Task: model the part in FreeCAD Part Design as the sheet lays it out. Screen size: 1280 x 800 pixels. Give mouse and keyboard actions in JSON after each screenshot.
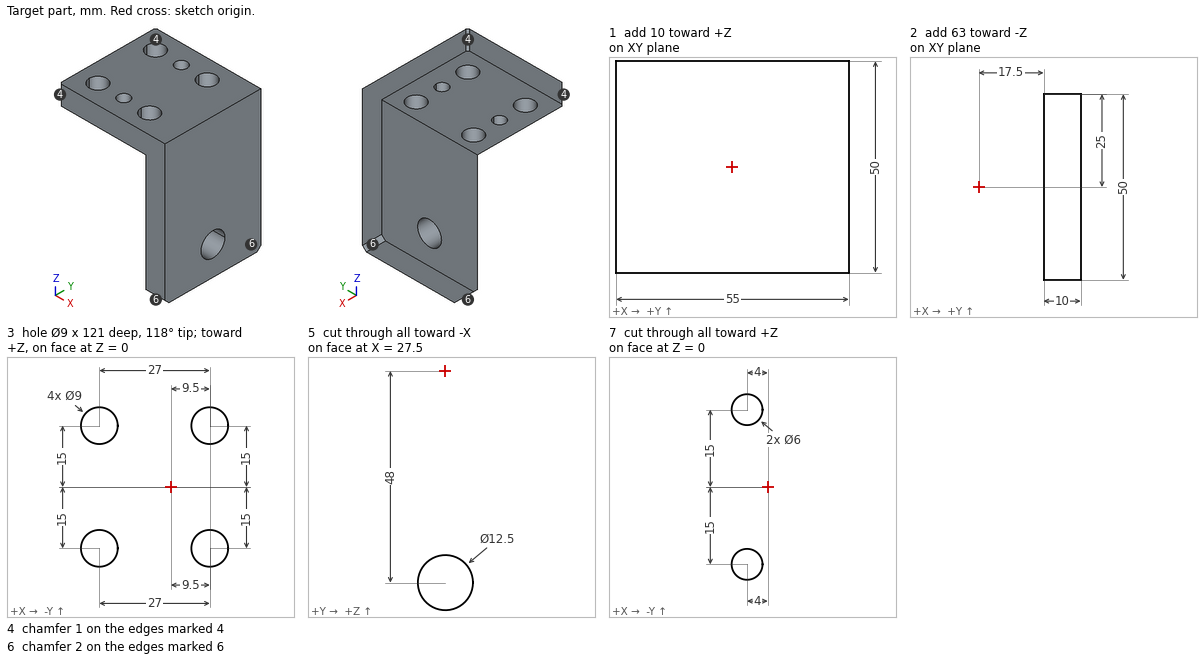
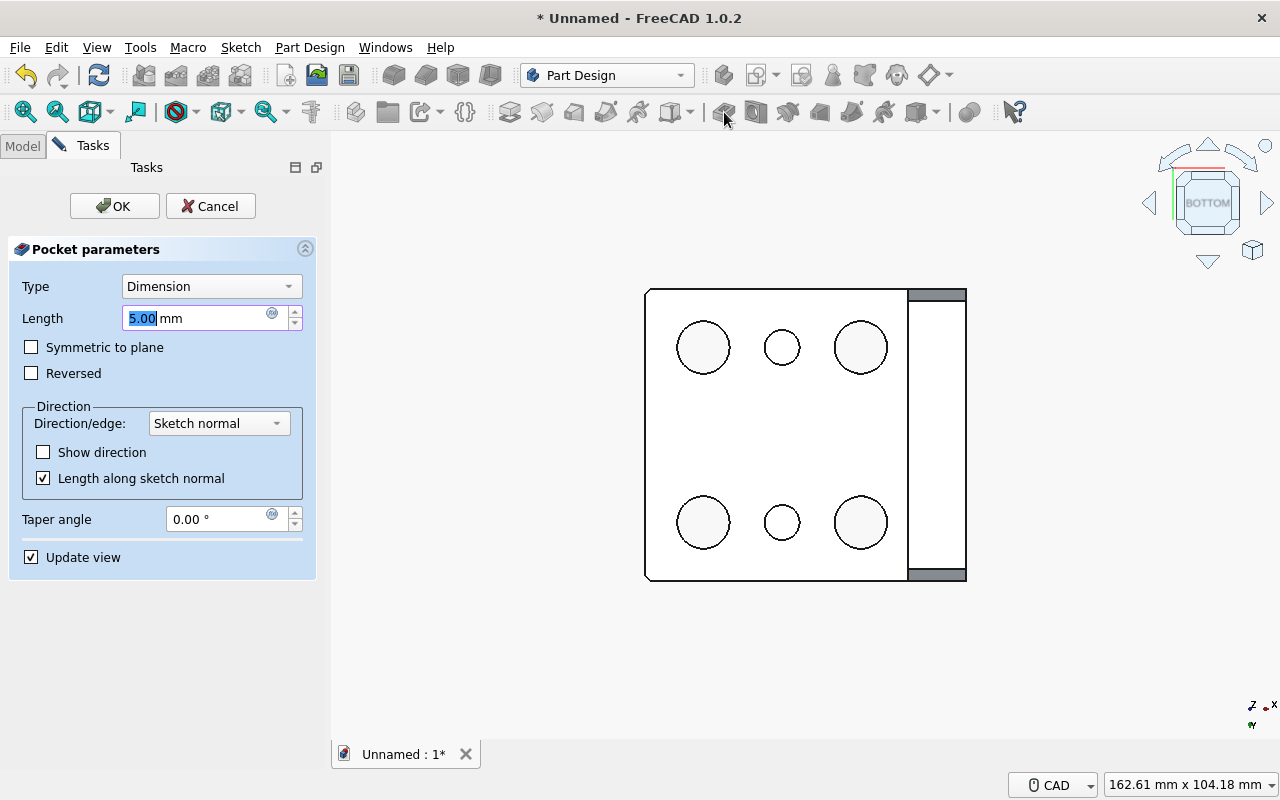
{"action": "left_click", "coordinate": [212, 286]}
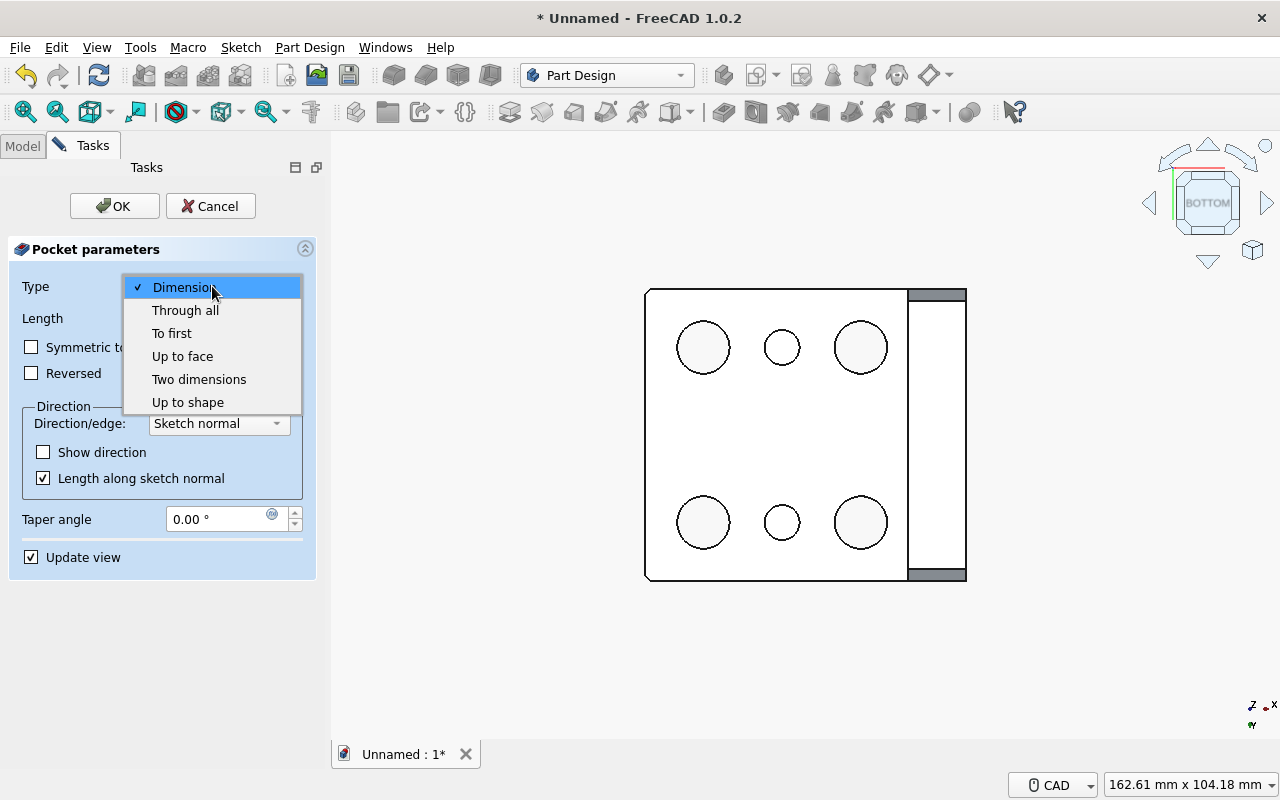
{"action": "left_click", "coordinate": [212, 310]}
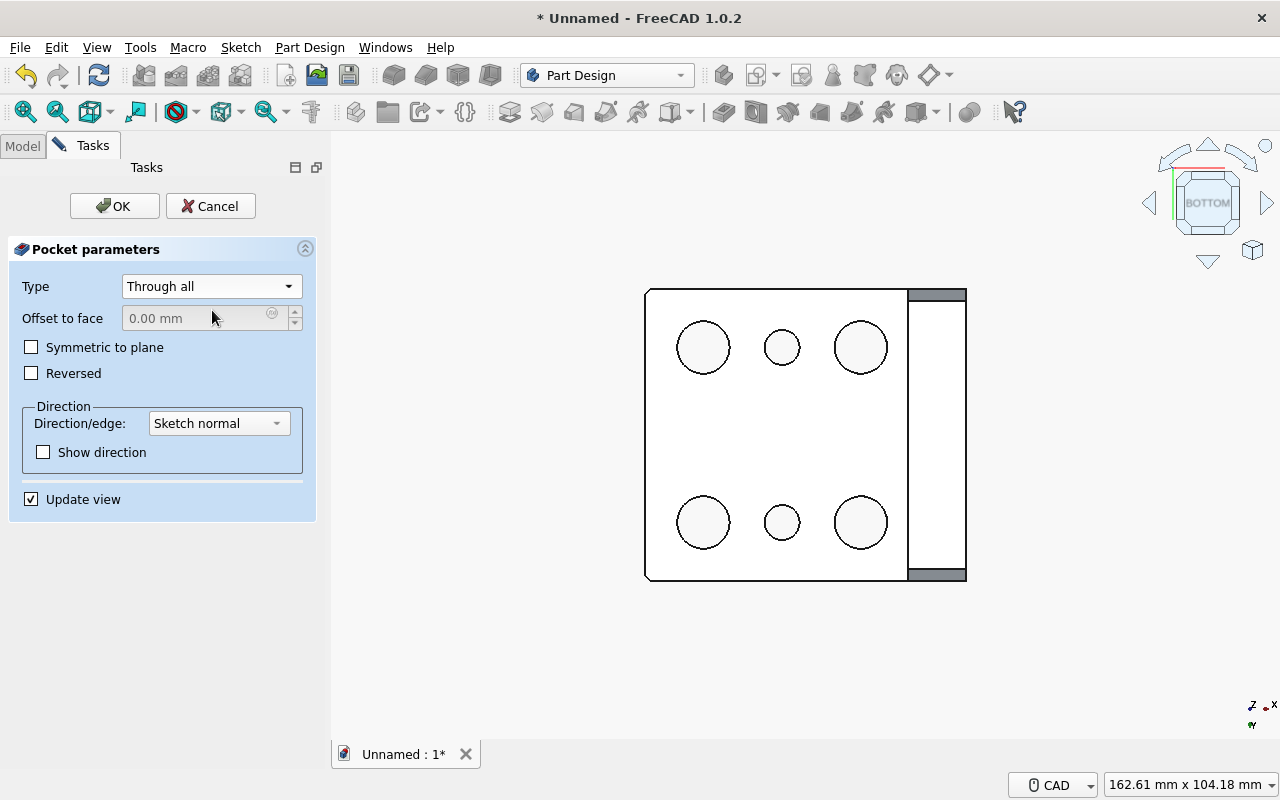
{"action": "left_click", "coordinate": [115, 206]}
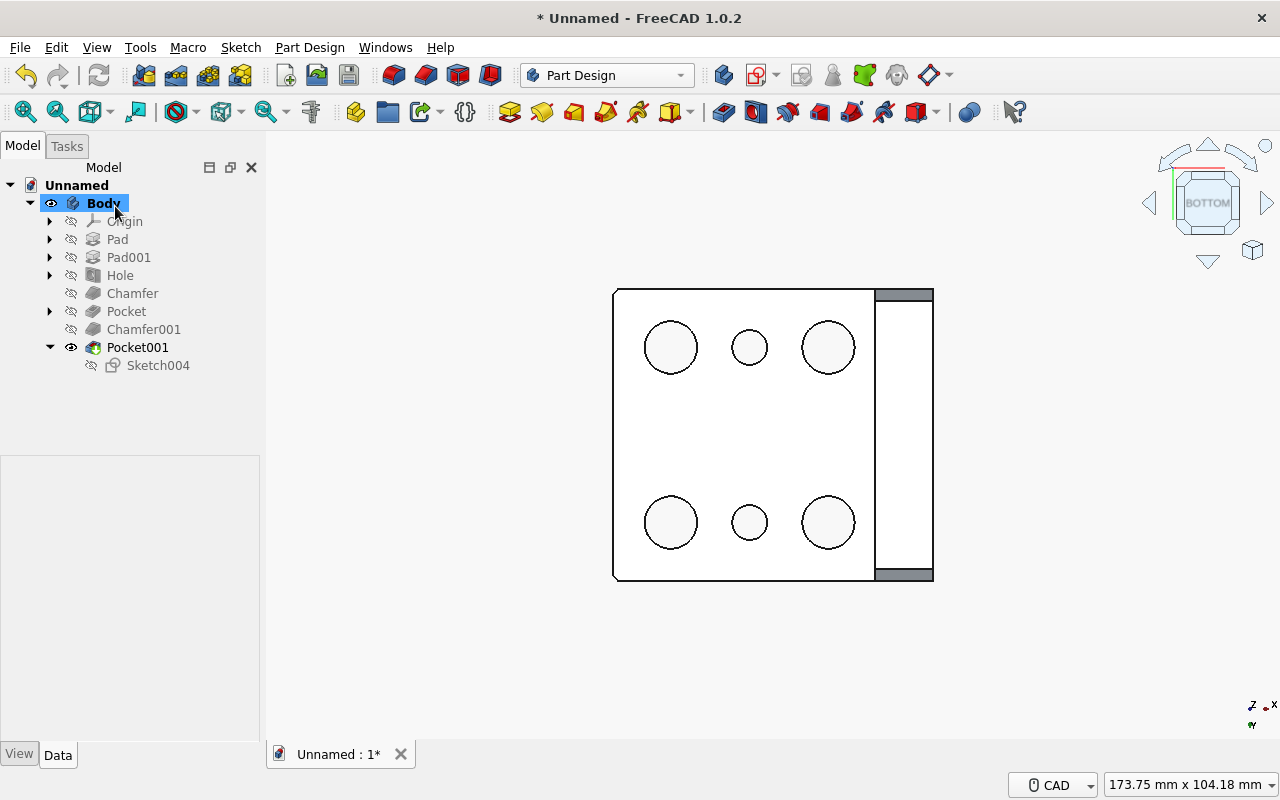
{"action": "key", "text": "0"}